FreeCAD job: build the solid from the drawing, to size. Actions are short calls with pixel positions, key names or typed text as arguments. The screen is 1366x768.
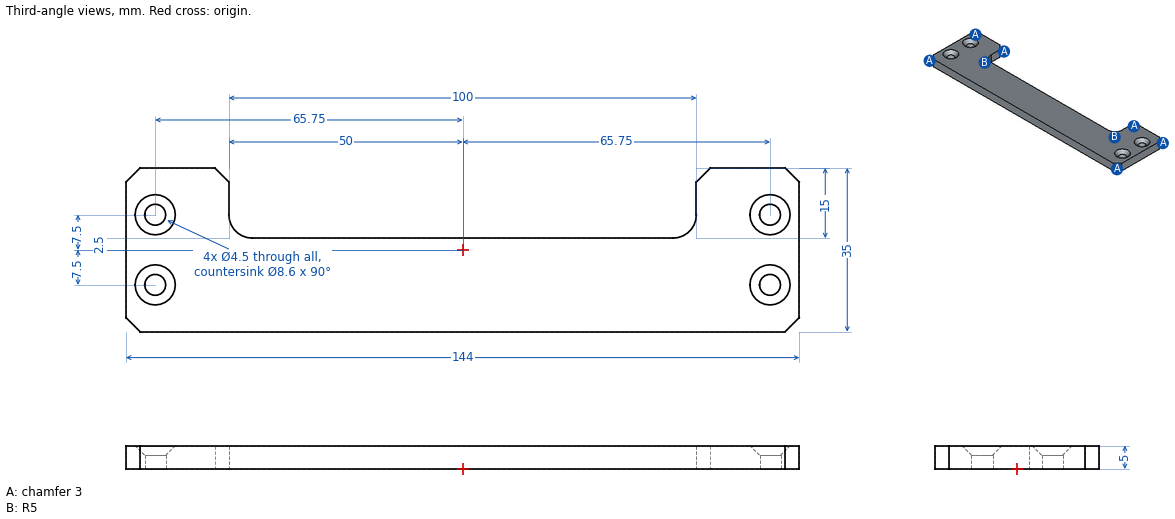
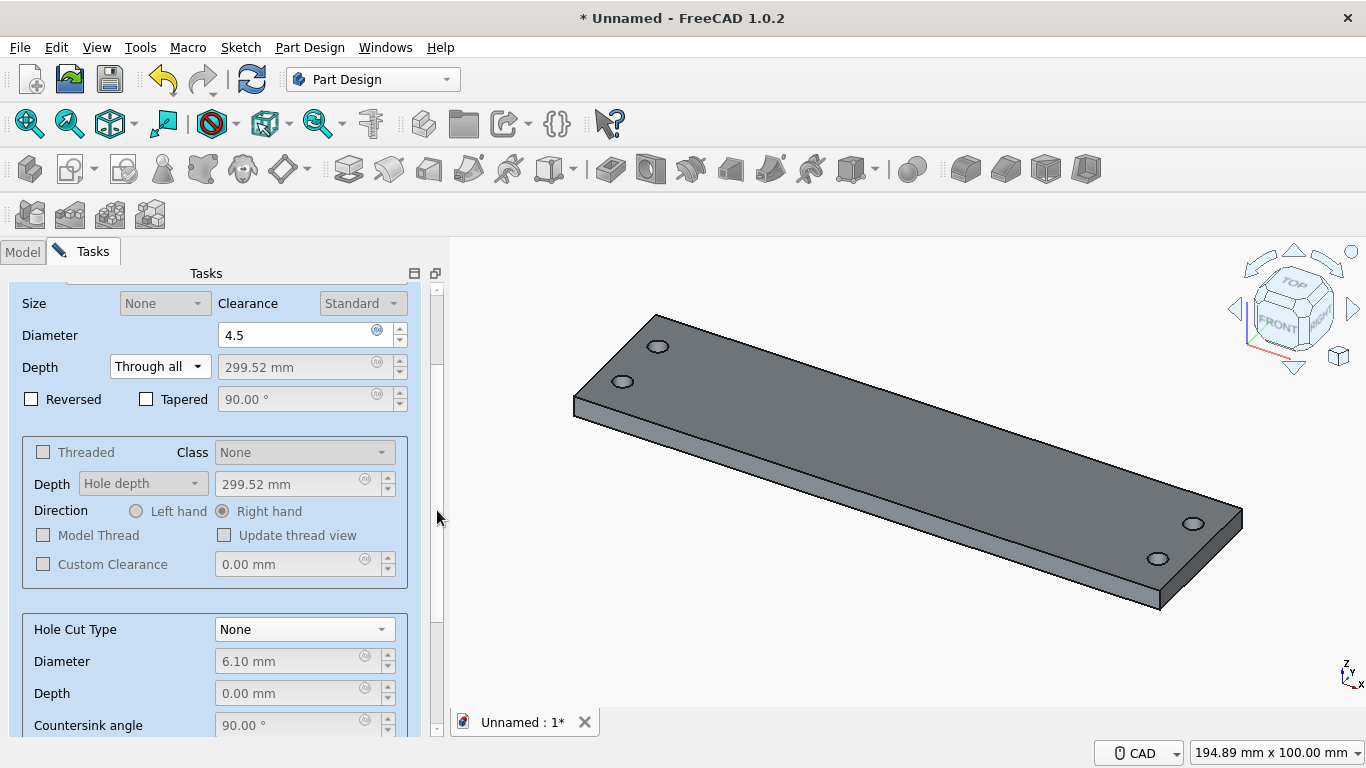
click(306, 630)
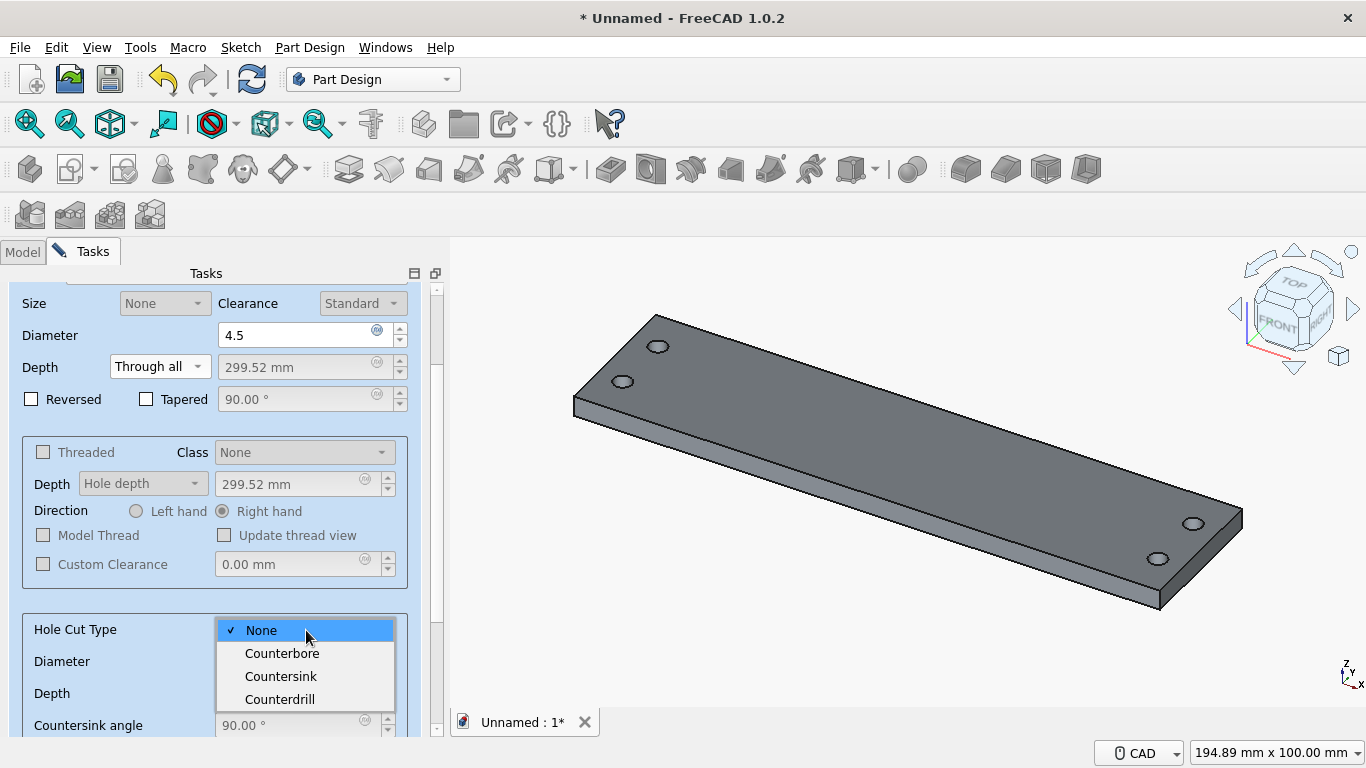
click(304, 676)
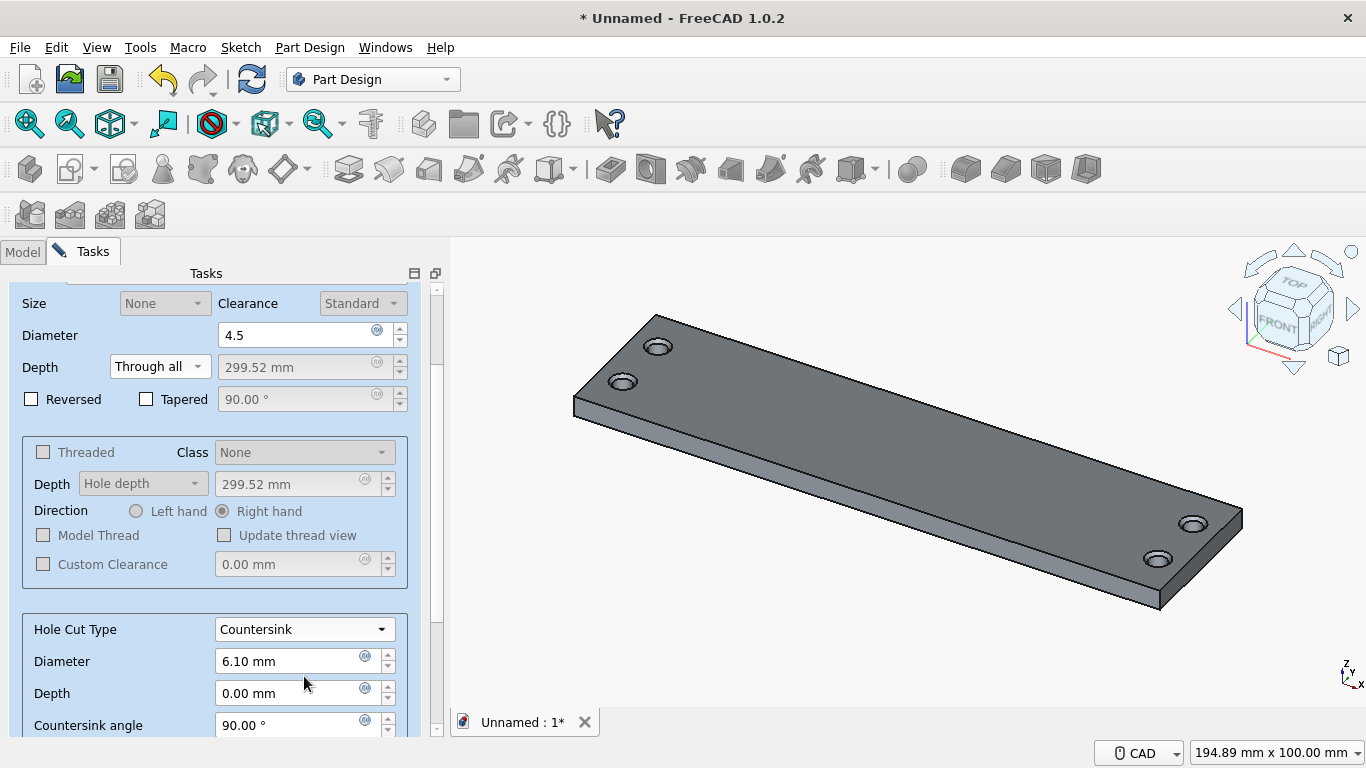
triple_click(298, 661)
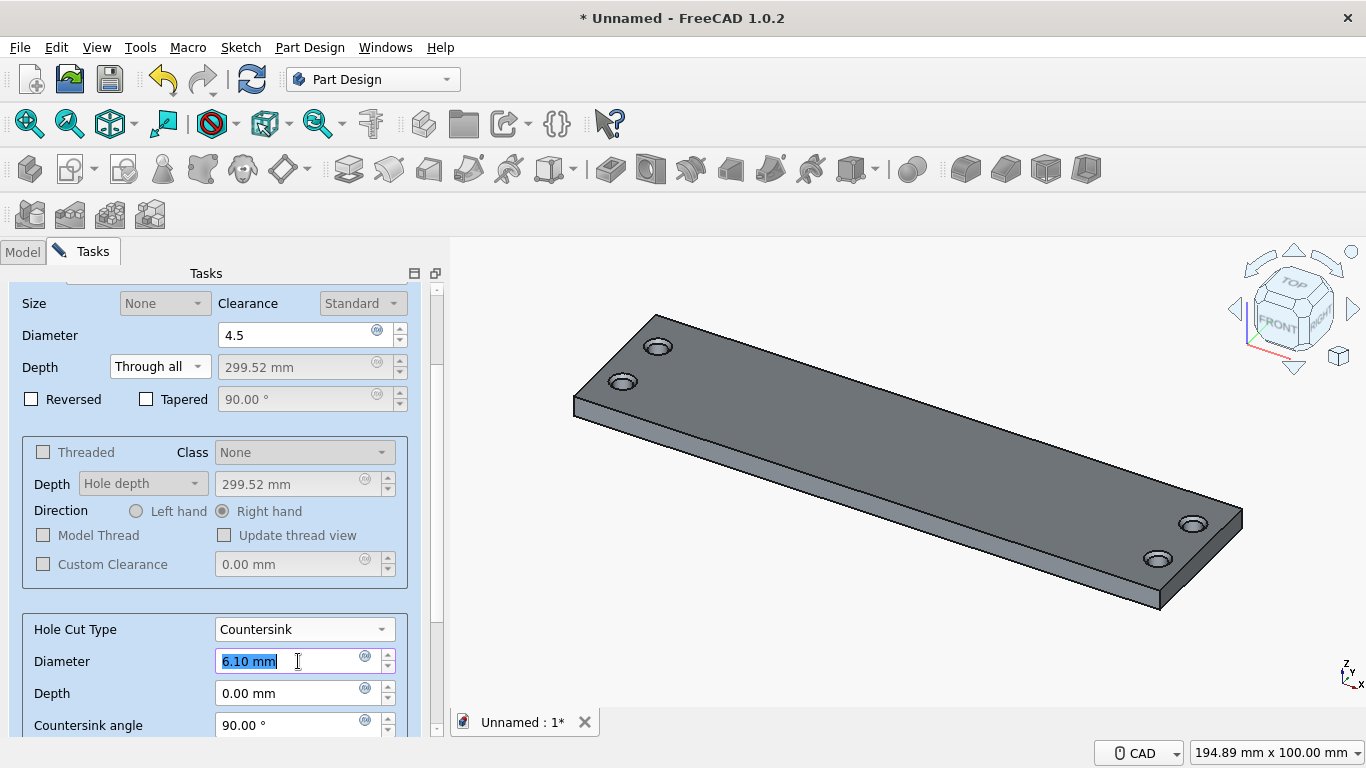
text(8.6)
key(Tab)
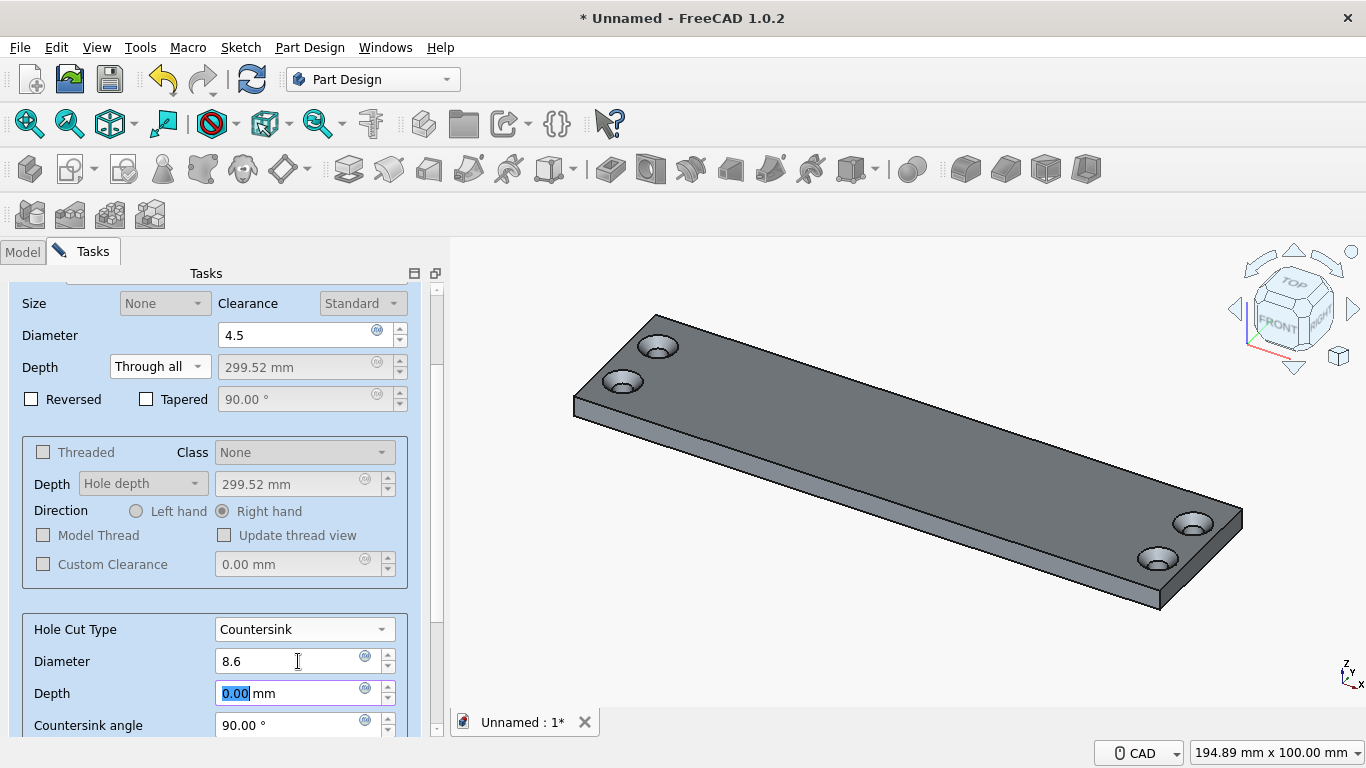
scroll(437, 510, up, 3)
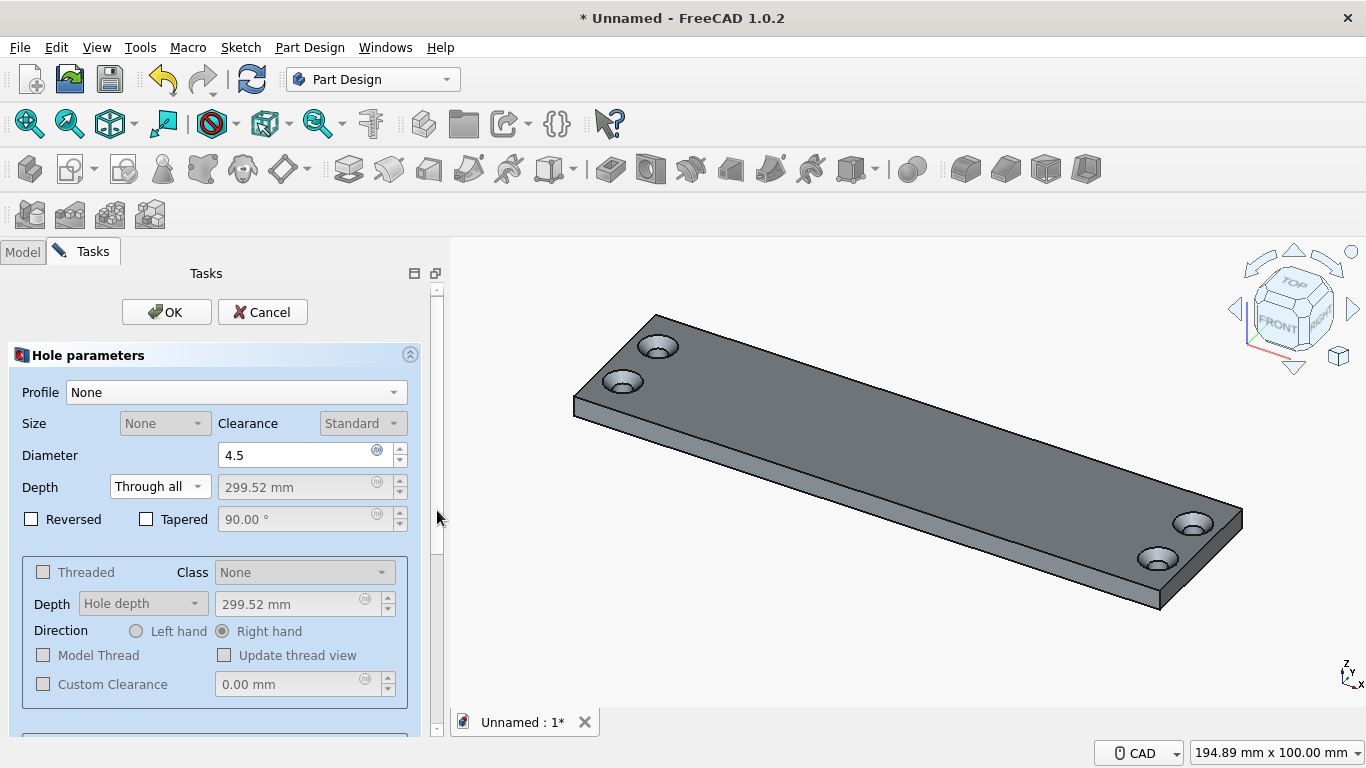
click(167, 312)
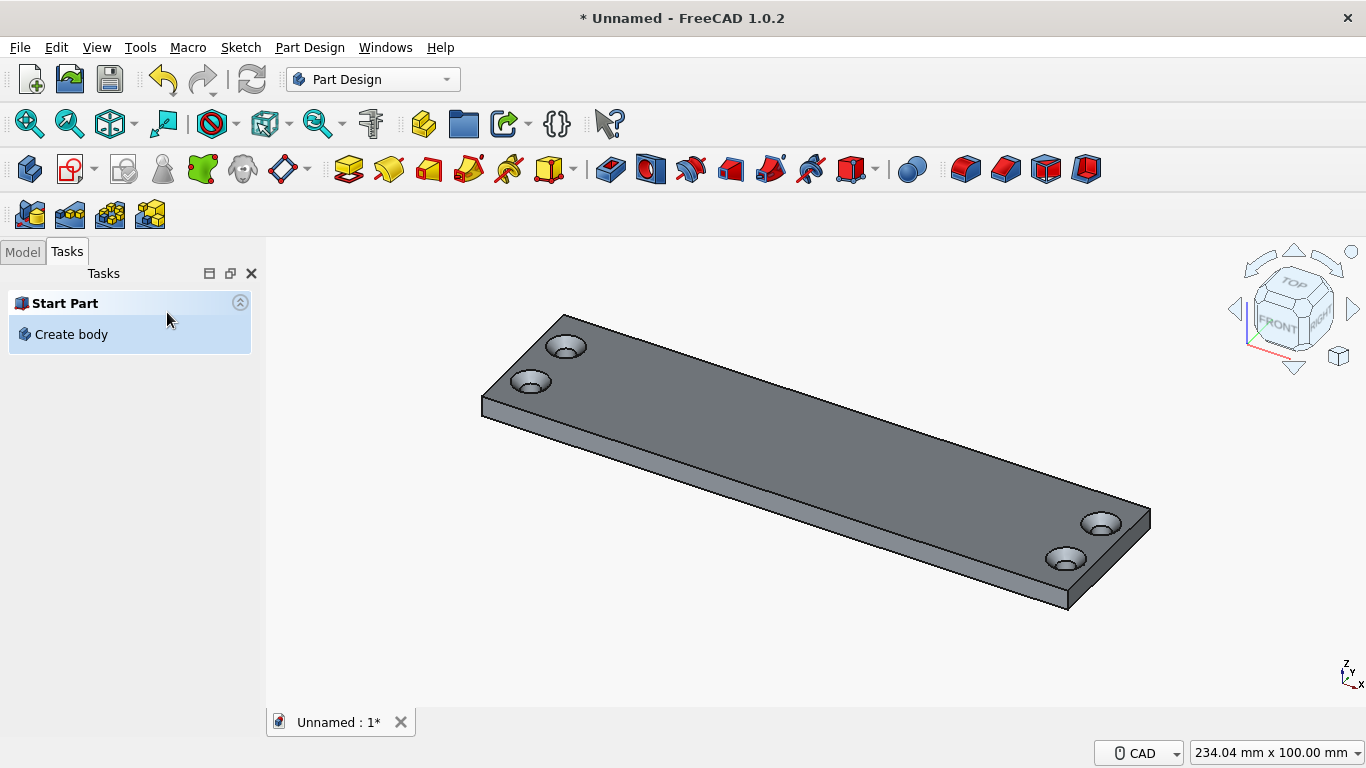
click(983, 507)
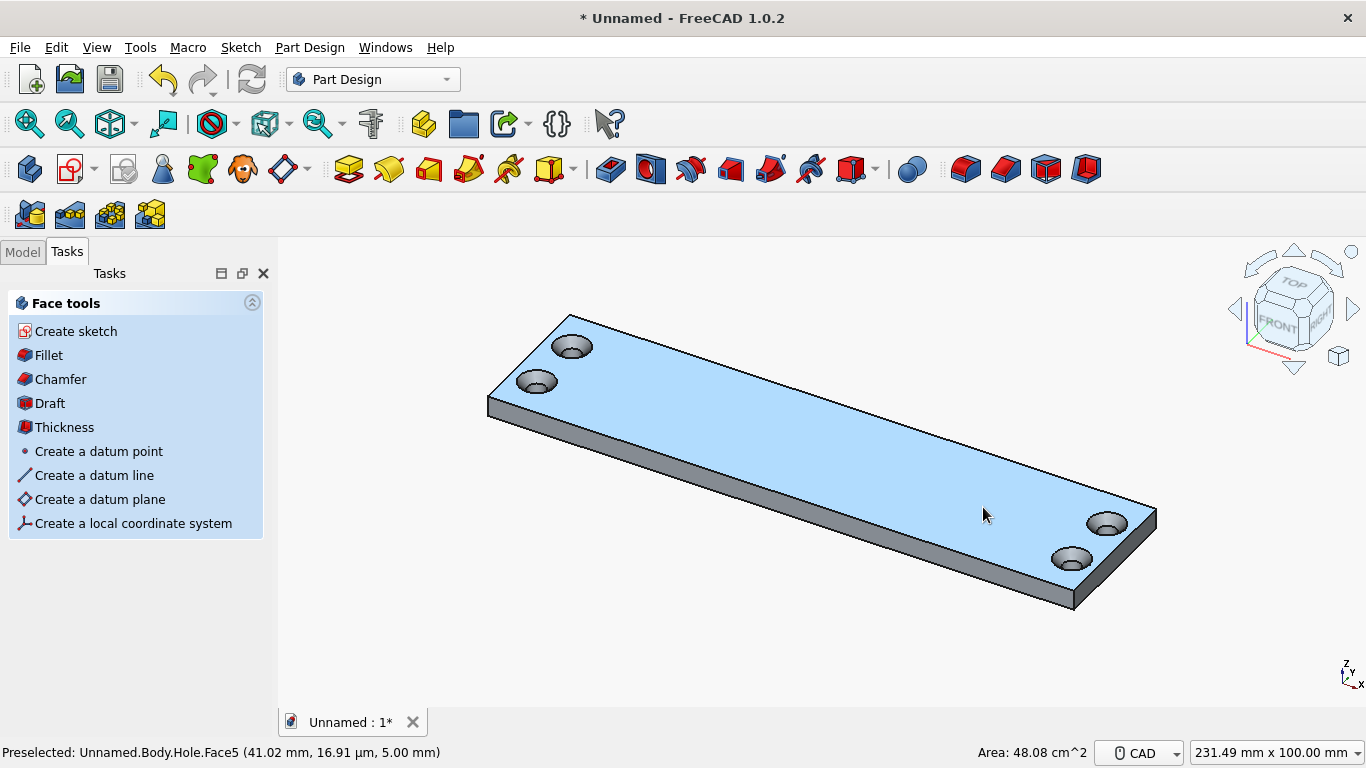
click(70, 170)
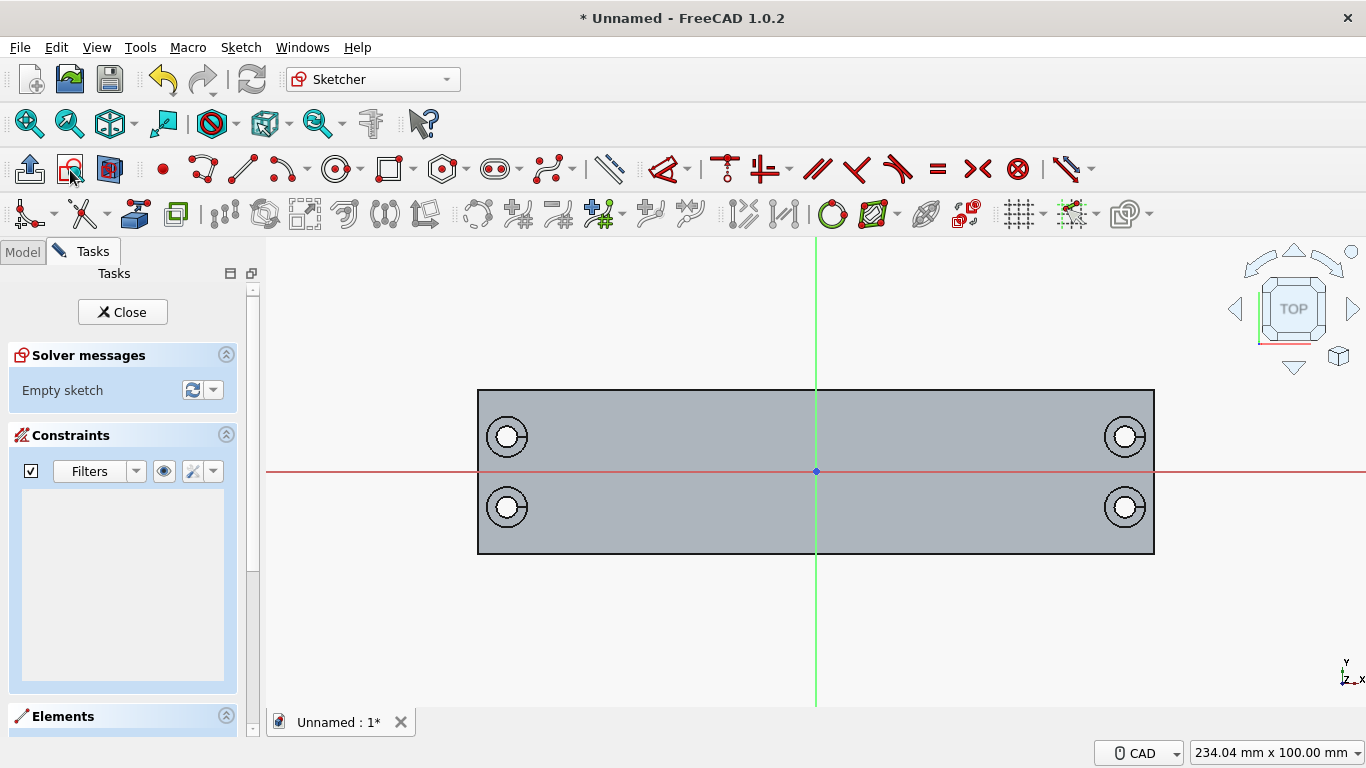
scroll(955, 347, up, 2)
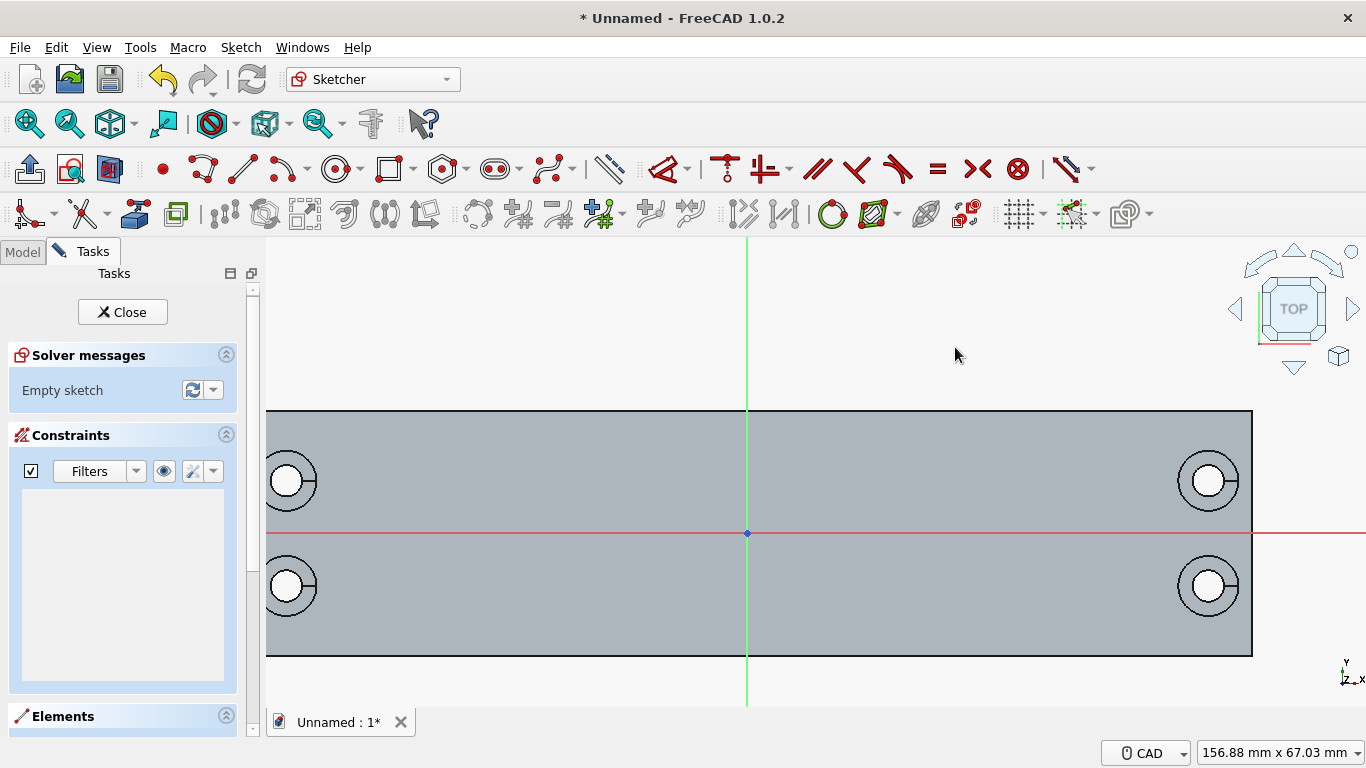
key(g)
key(r)